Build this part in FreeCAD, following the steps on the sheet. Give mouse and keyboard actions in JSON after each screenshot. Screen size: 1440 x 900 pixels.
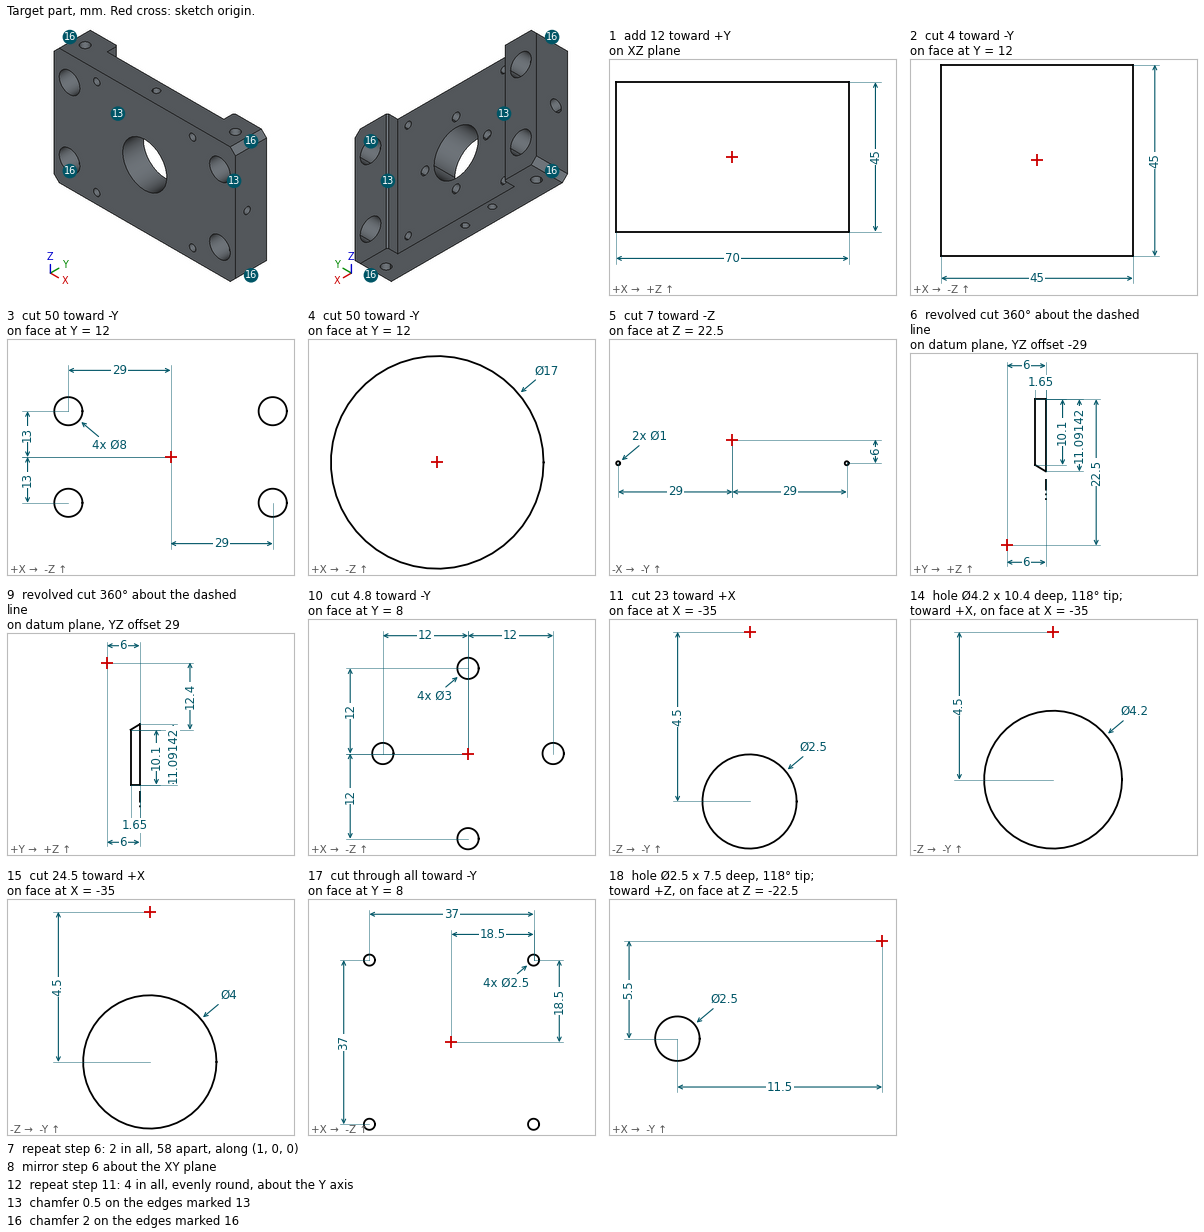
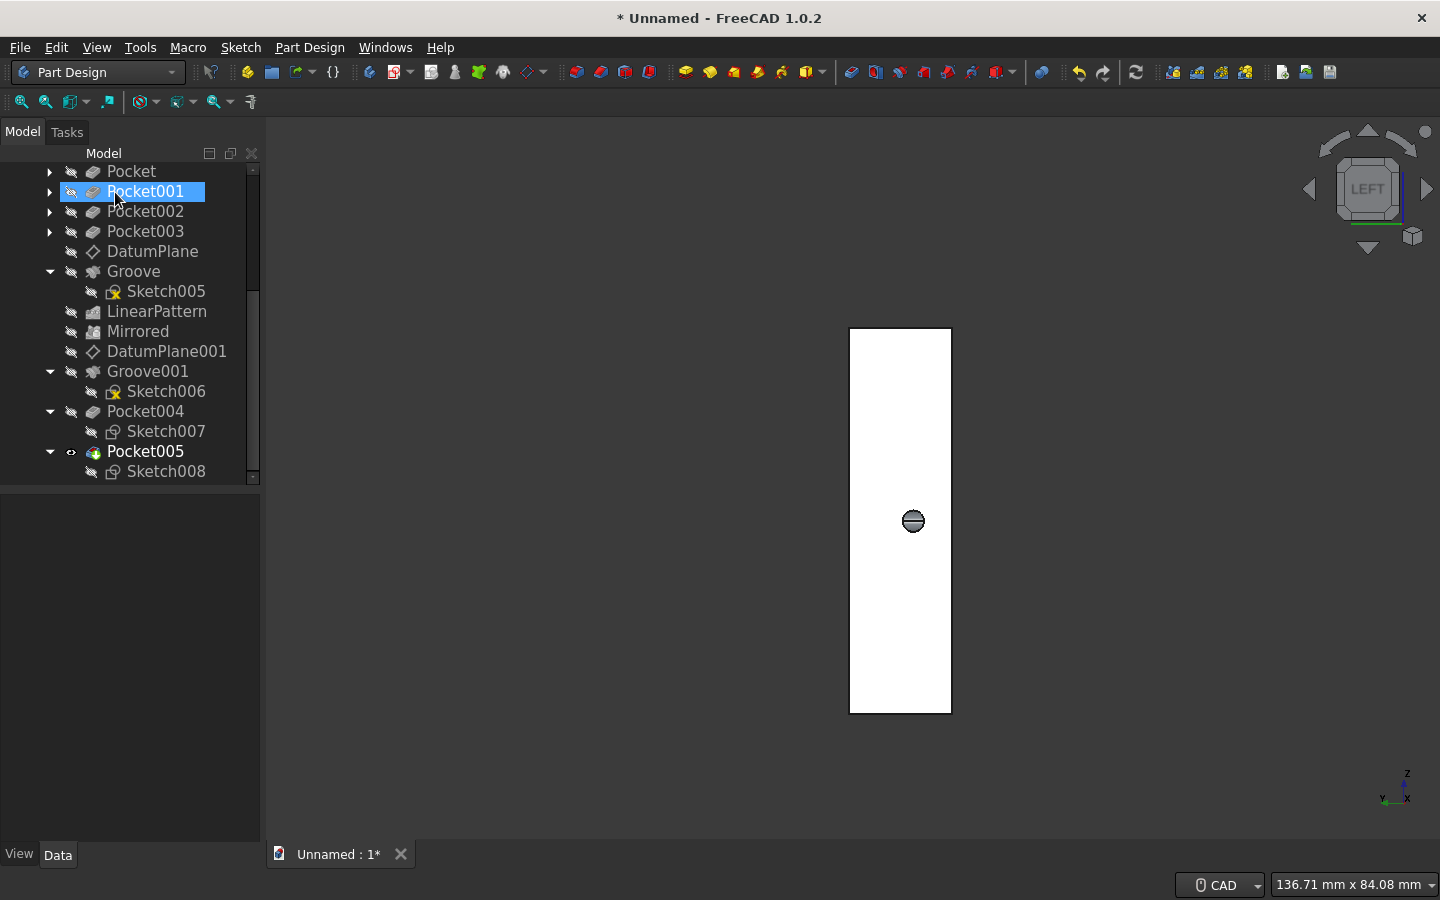
{"action": "left_click", "coordinate": [116, 452]}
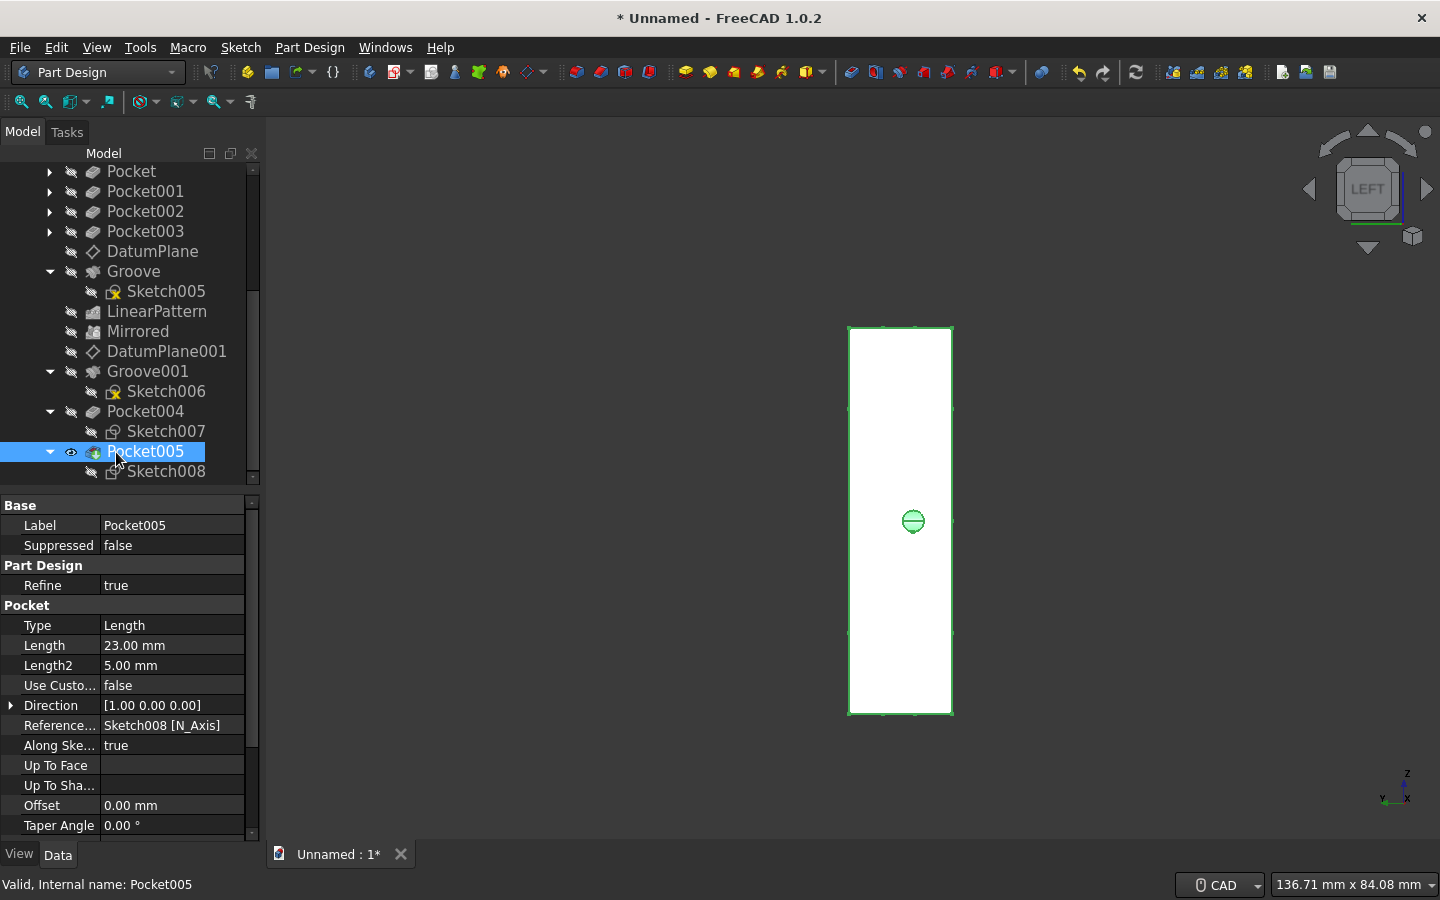
{"action": "left_click", "coordinate": [1222, 72]}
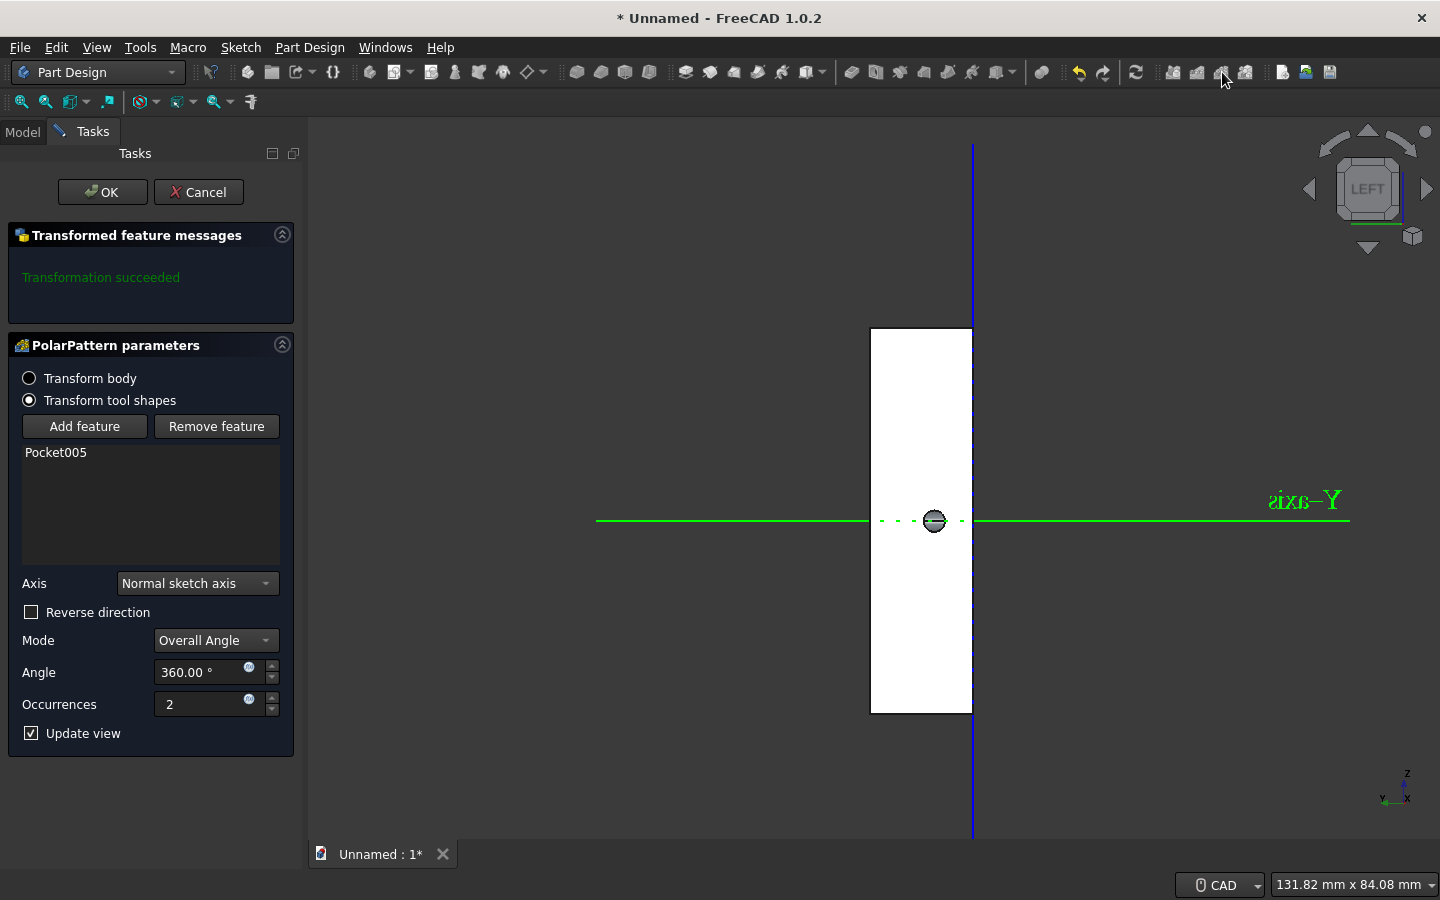
{"action": "left_click", "coordinate": [198, 584]}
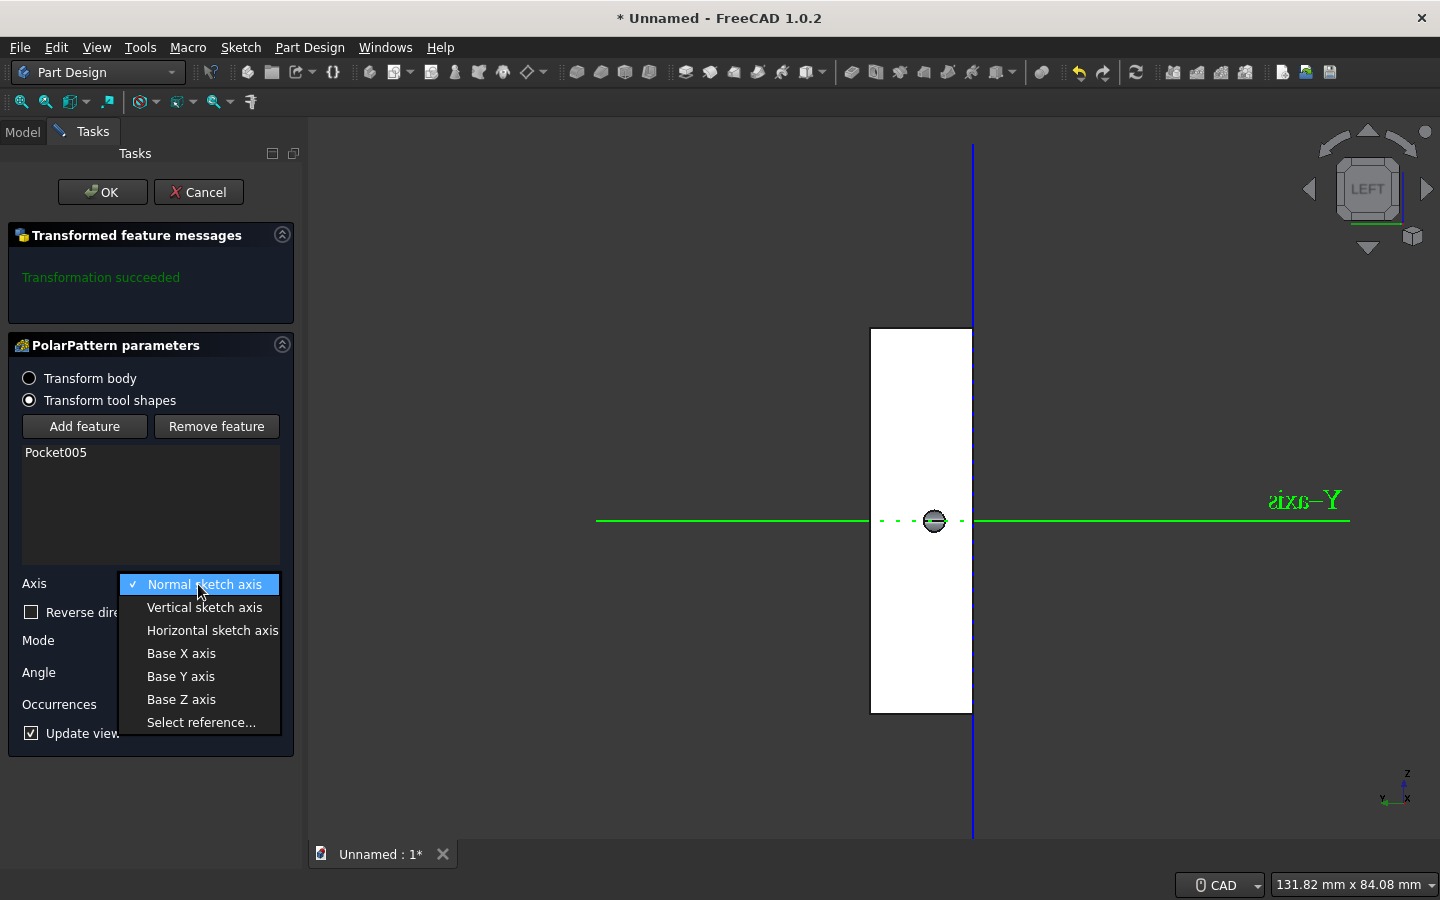
{"action": "left_click", "coordinate": [198, 676]}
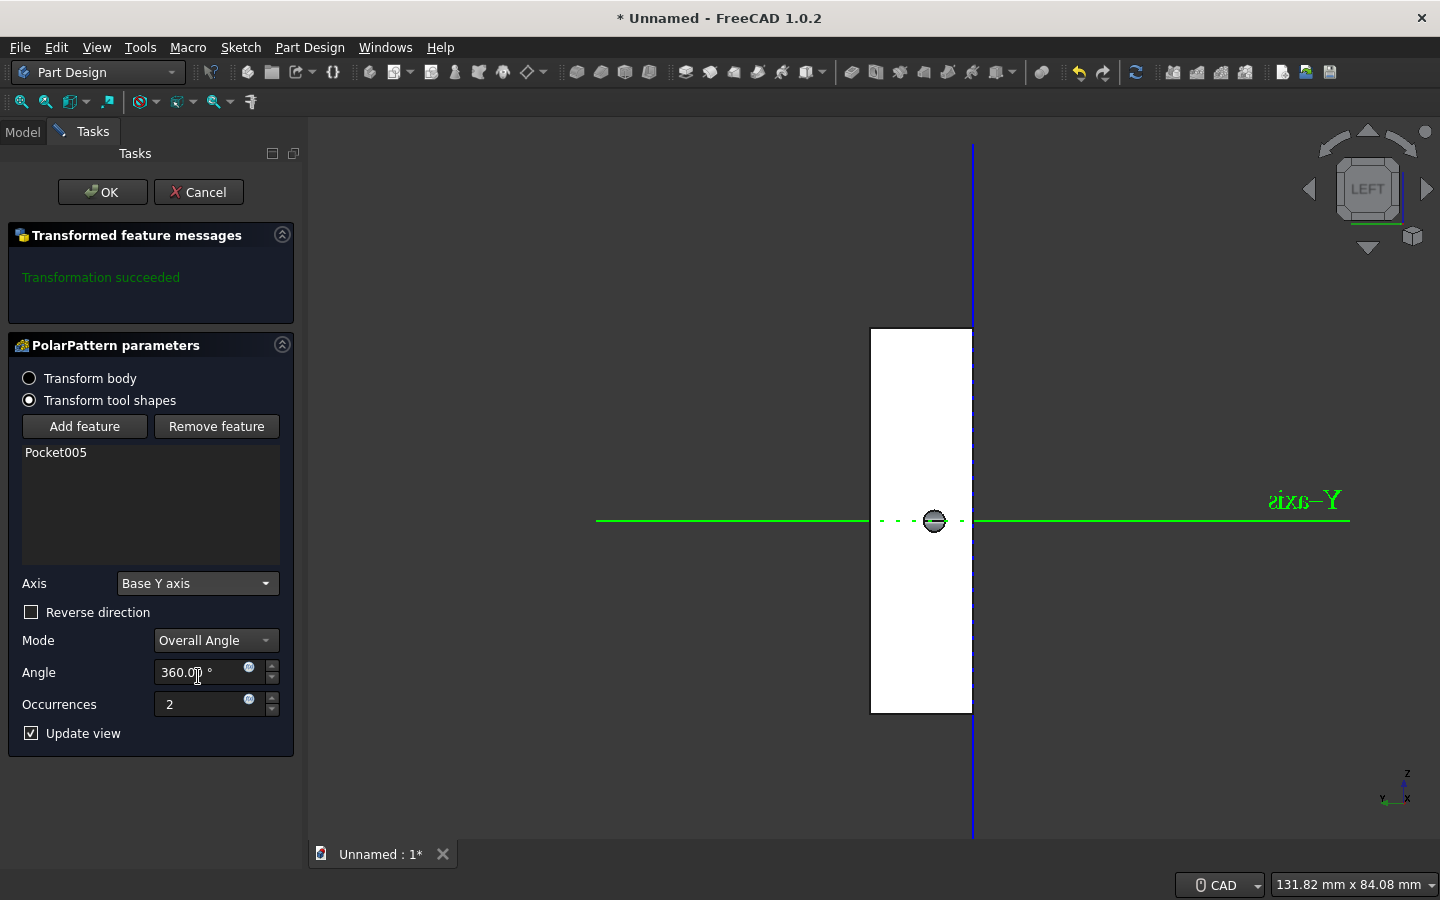
{"action": "triple_click", "coordinate": [209, 704]}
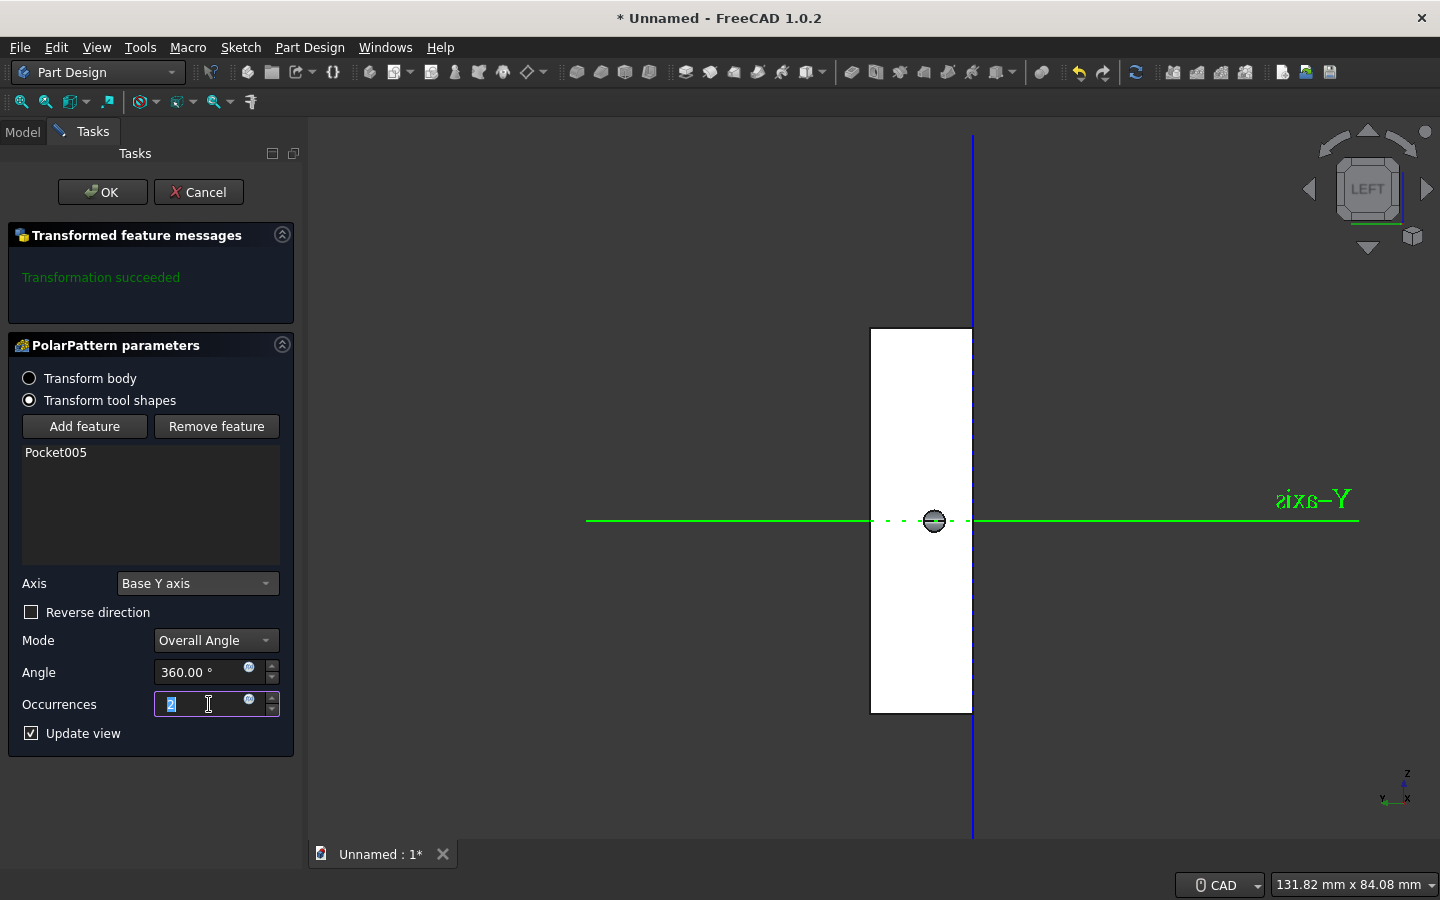
{"action": "type", "text": "4"}
{"action": "key", "text": "Tab"}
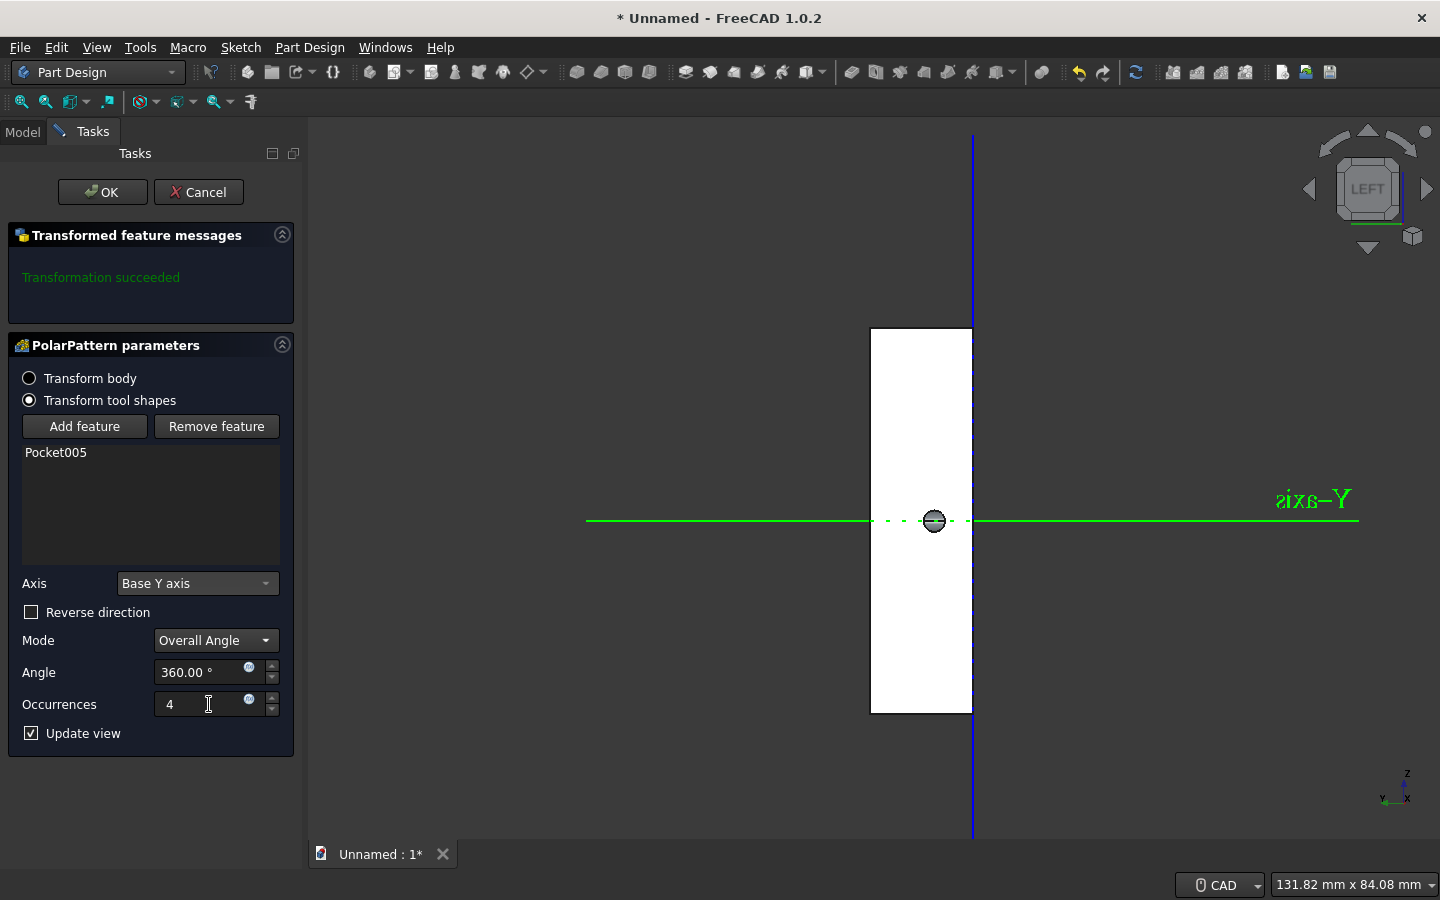
{"action": "left_click", "coordinate": [103, 192]}